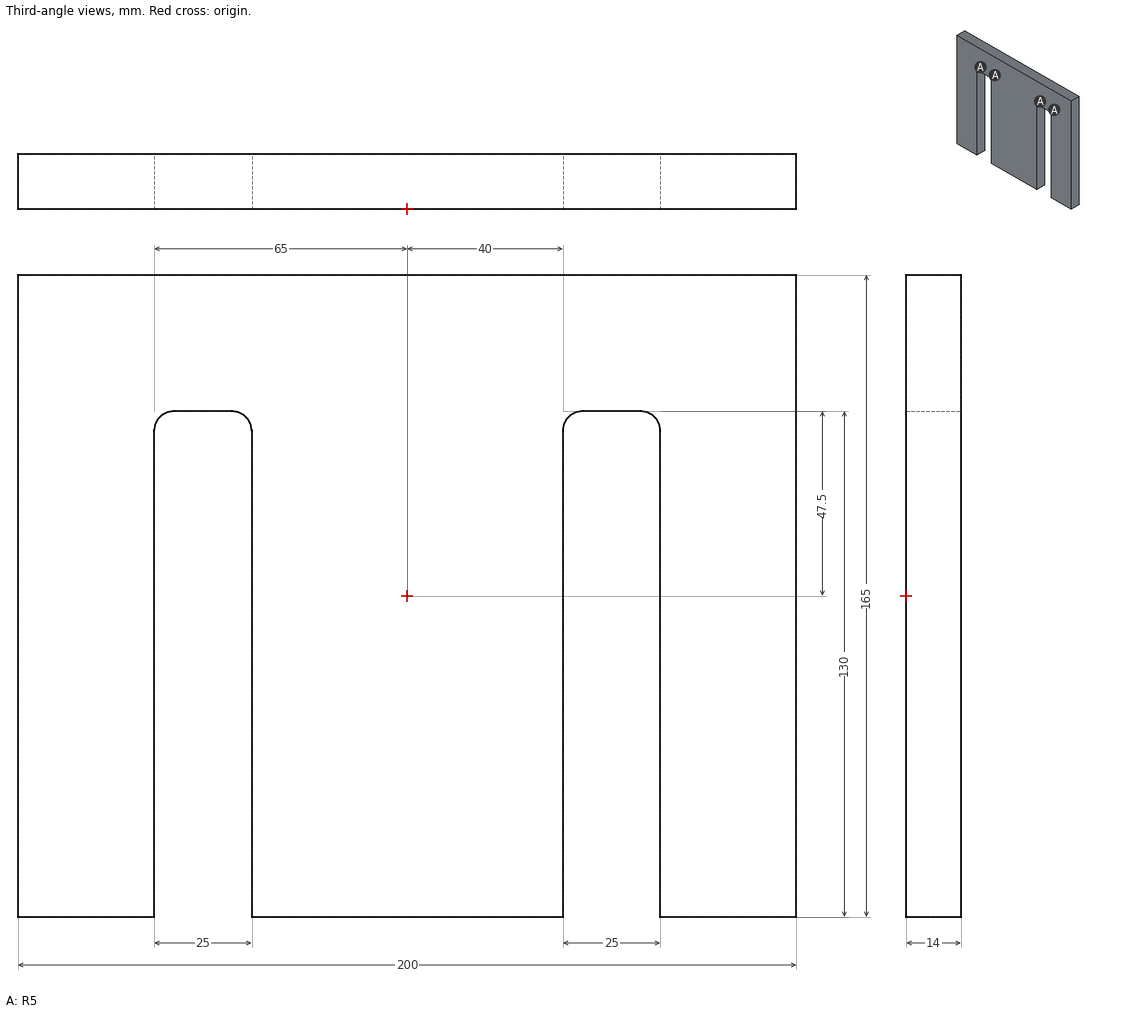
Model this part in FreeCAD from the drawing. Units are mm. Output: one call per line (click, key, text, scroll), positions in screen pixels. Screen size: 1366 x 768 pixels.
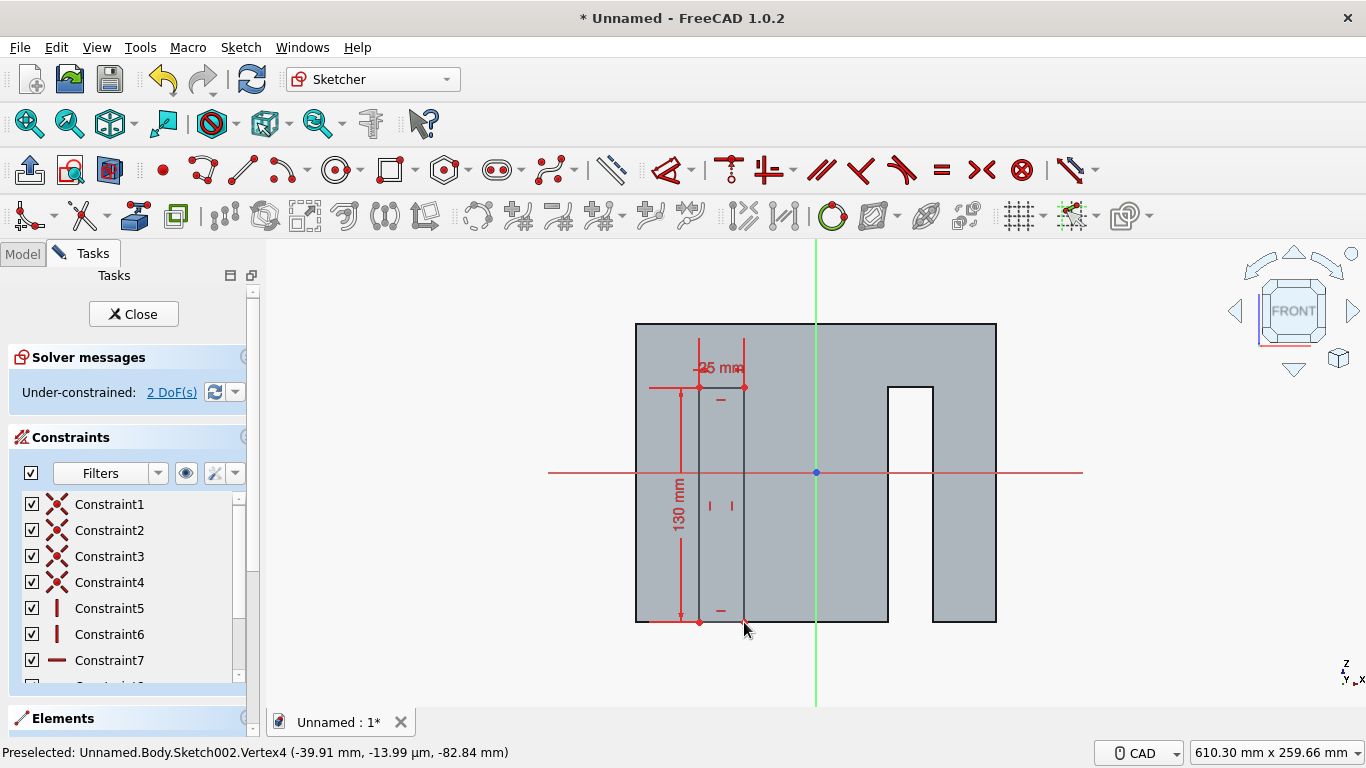
click(666, 170)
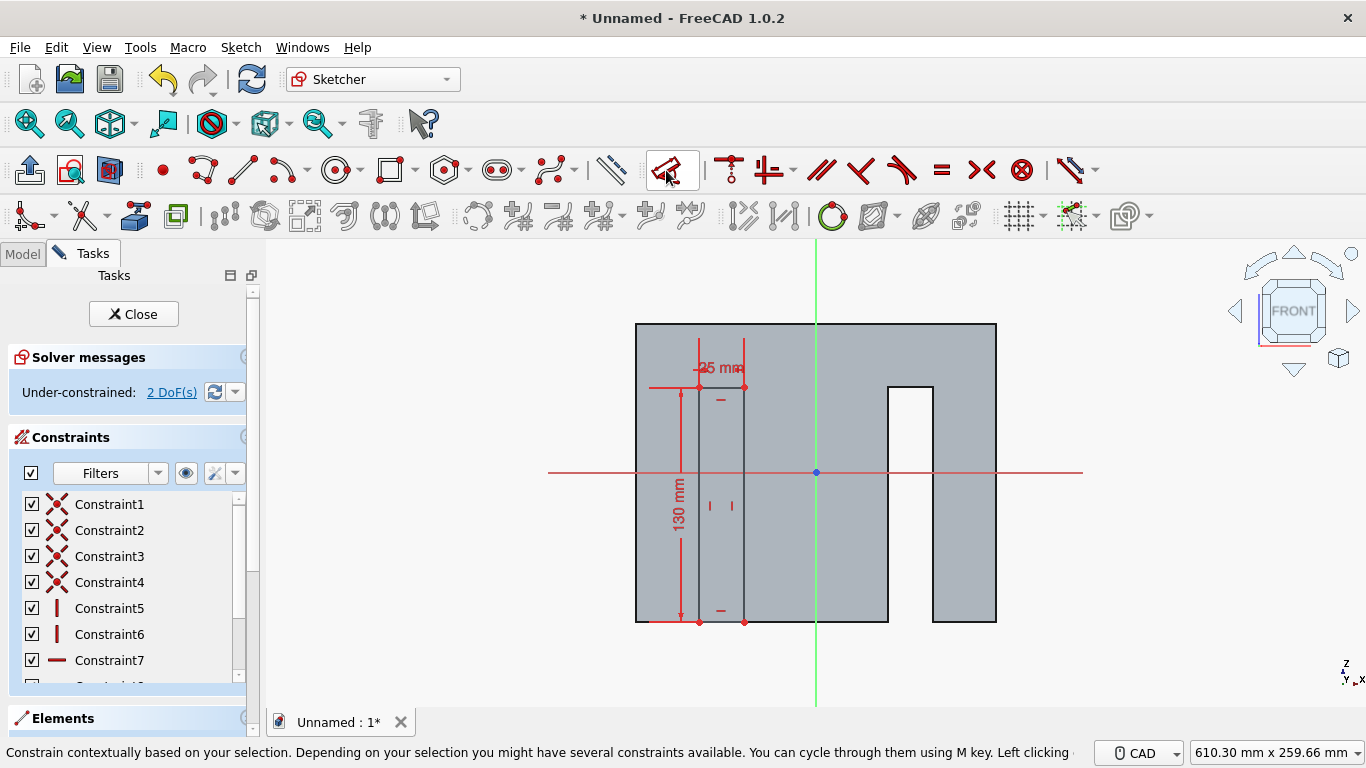
click(699, 388)
click(758, 354)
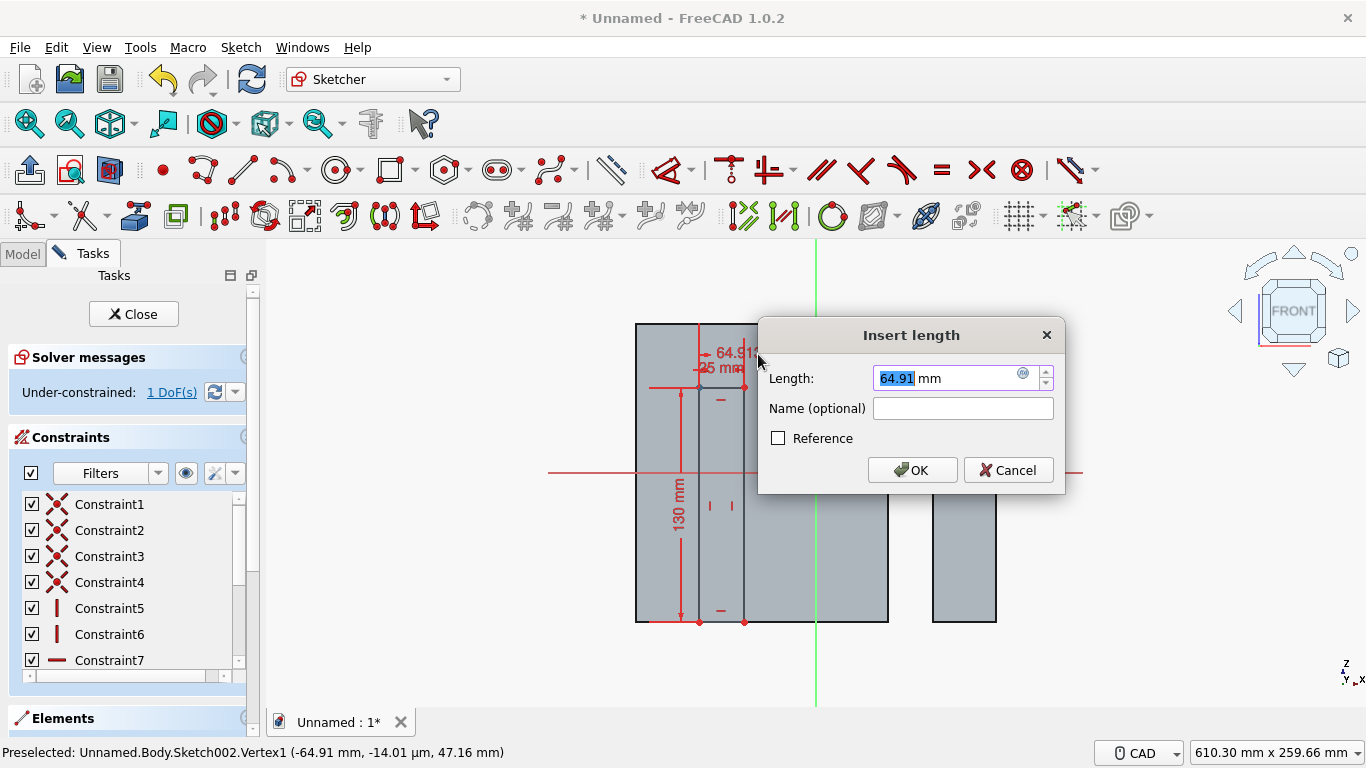
text(65)
key(Return)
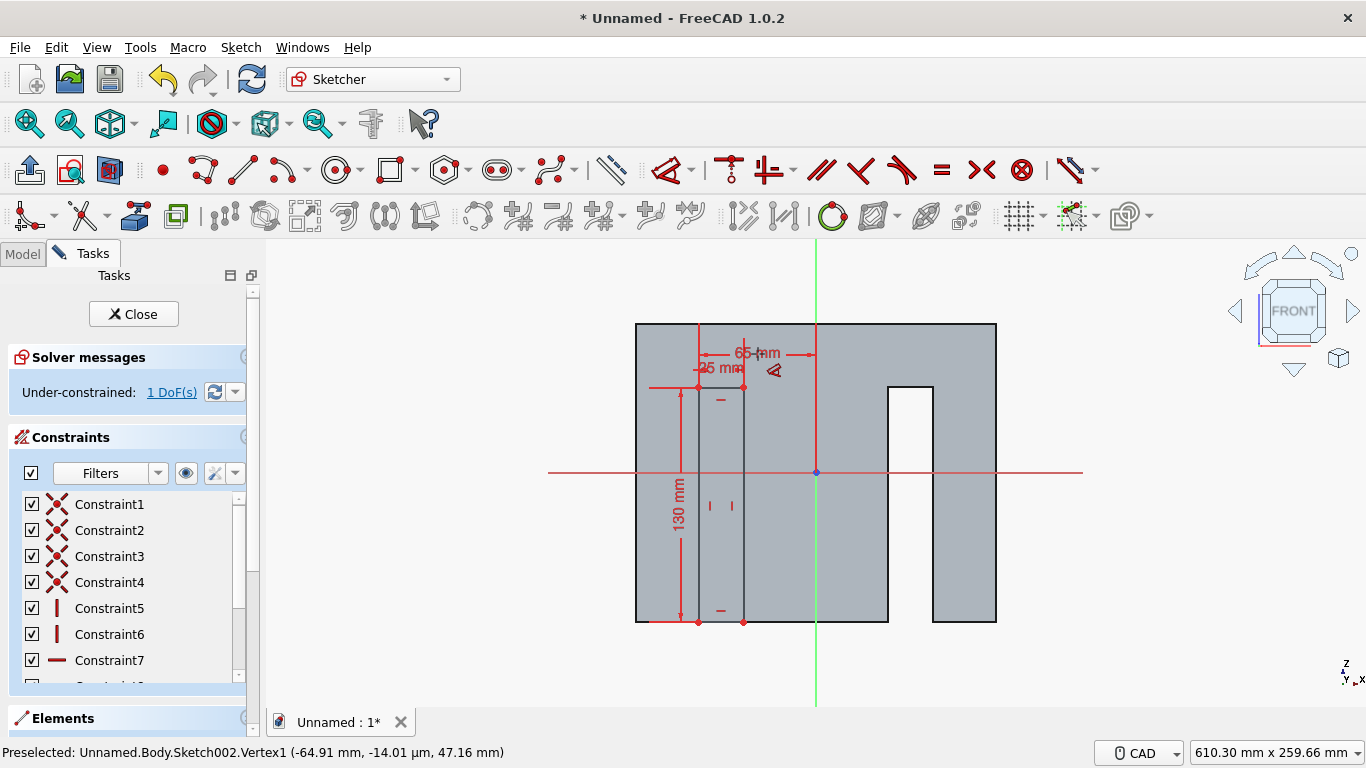
click(699, 388)
click(850, 430)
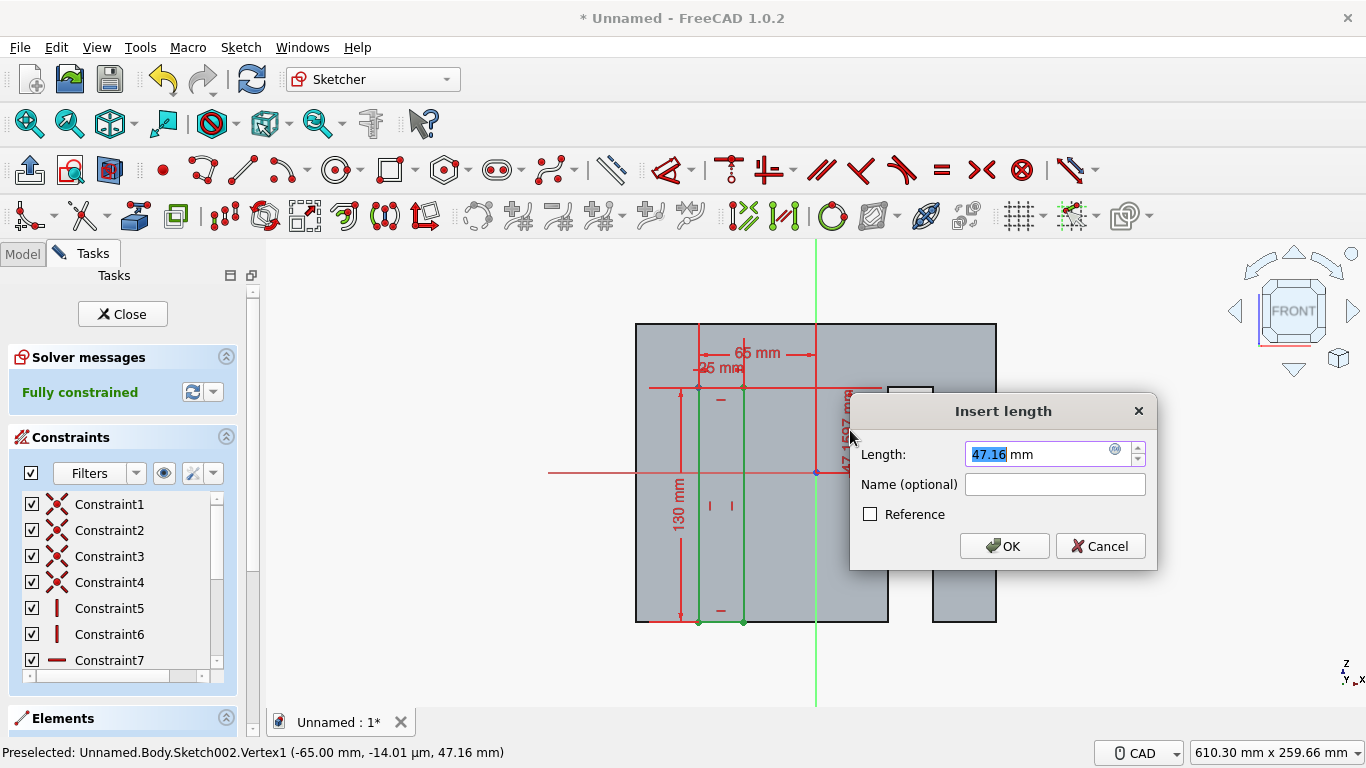
text(47.5)
key(Return)
key(Escape)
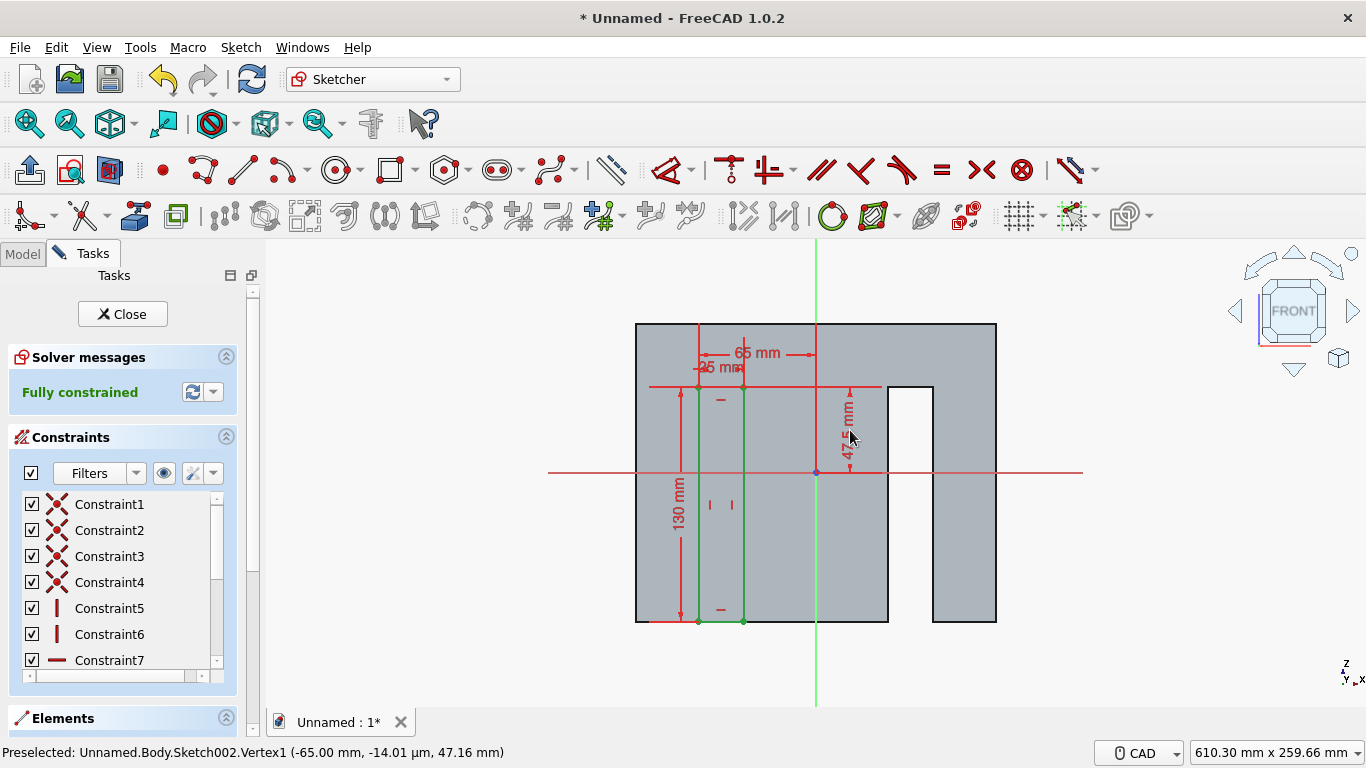
click(123, 314)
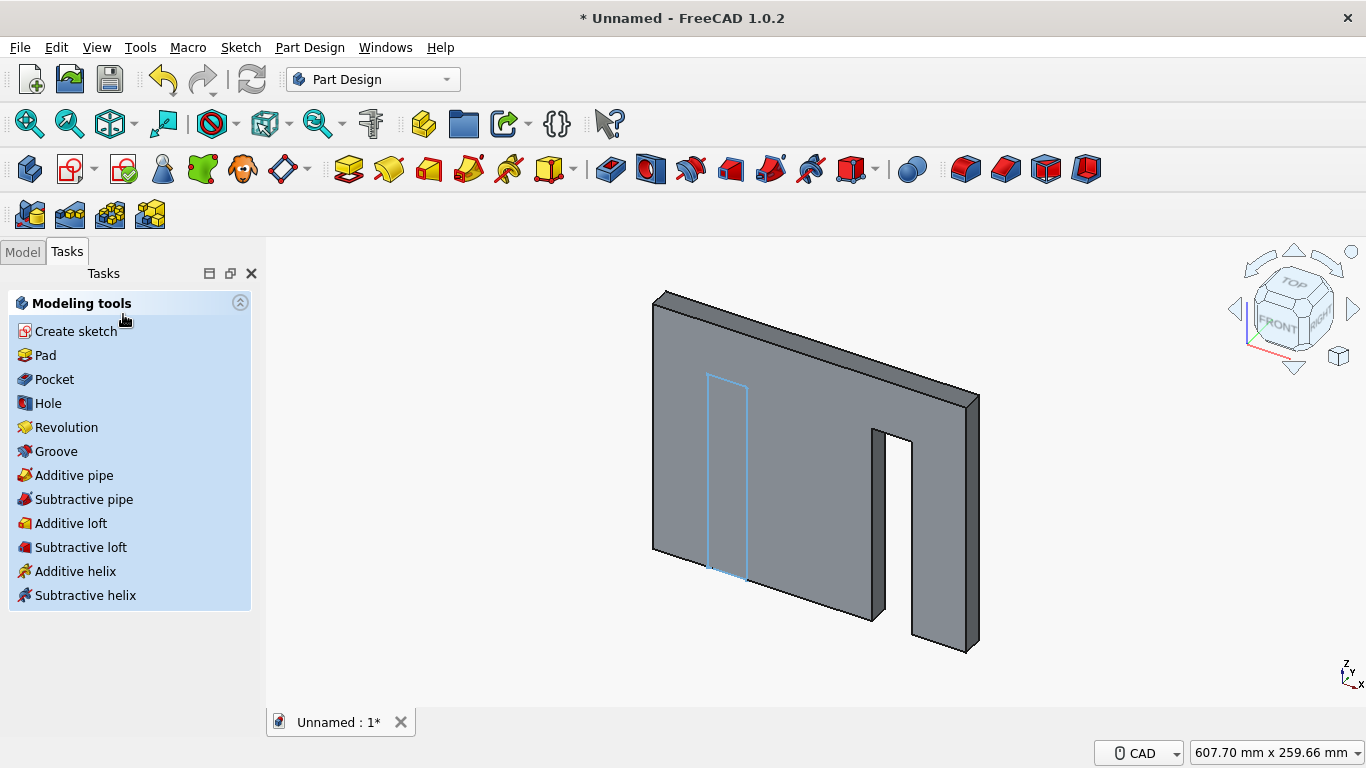
click(612, 170)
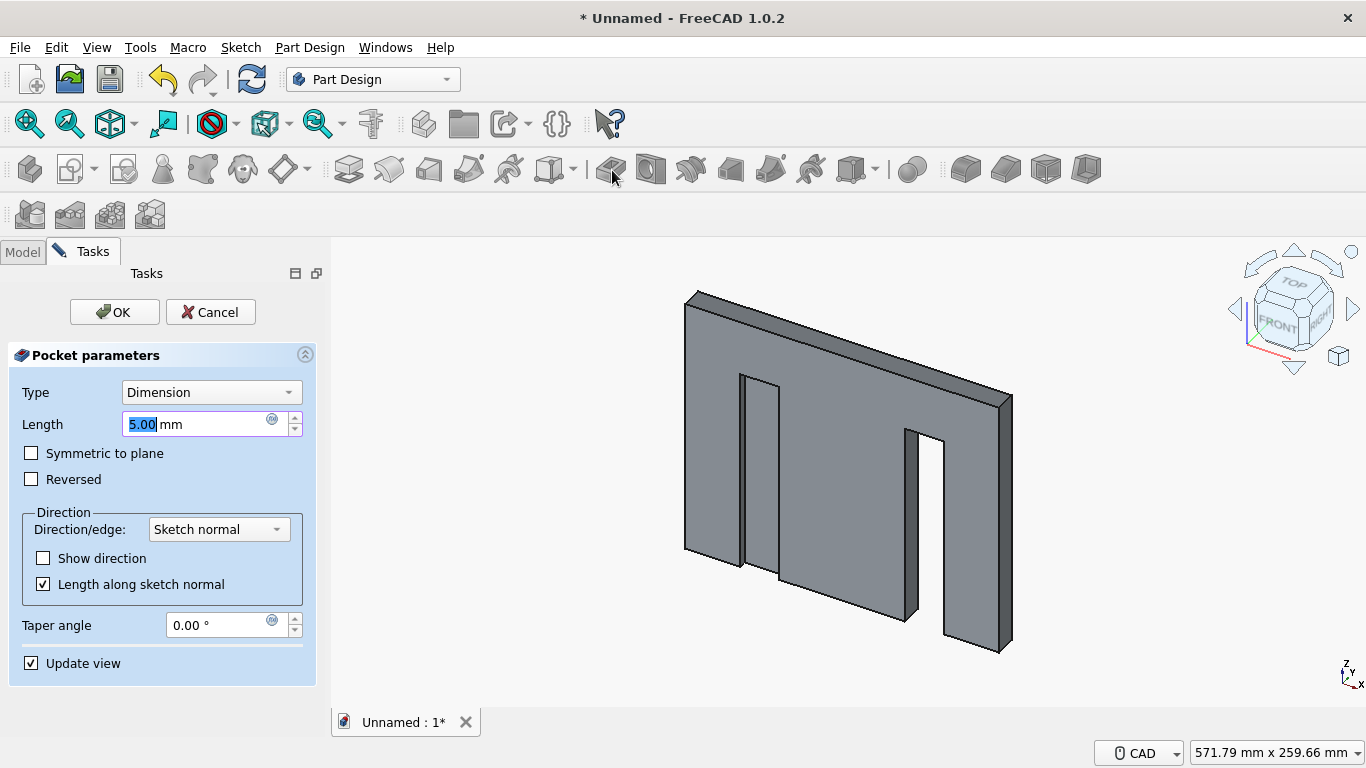
click(212, 392)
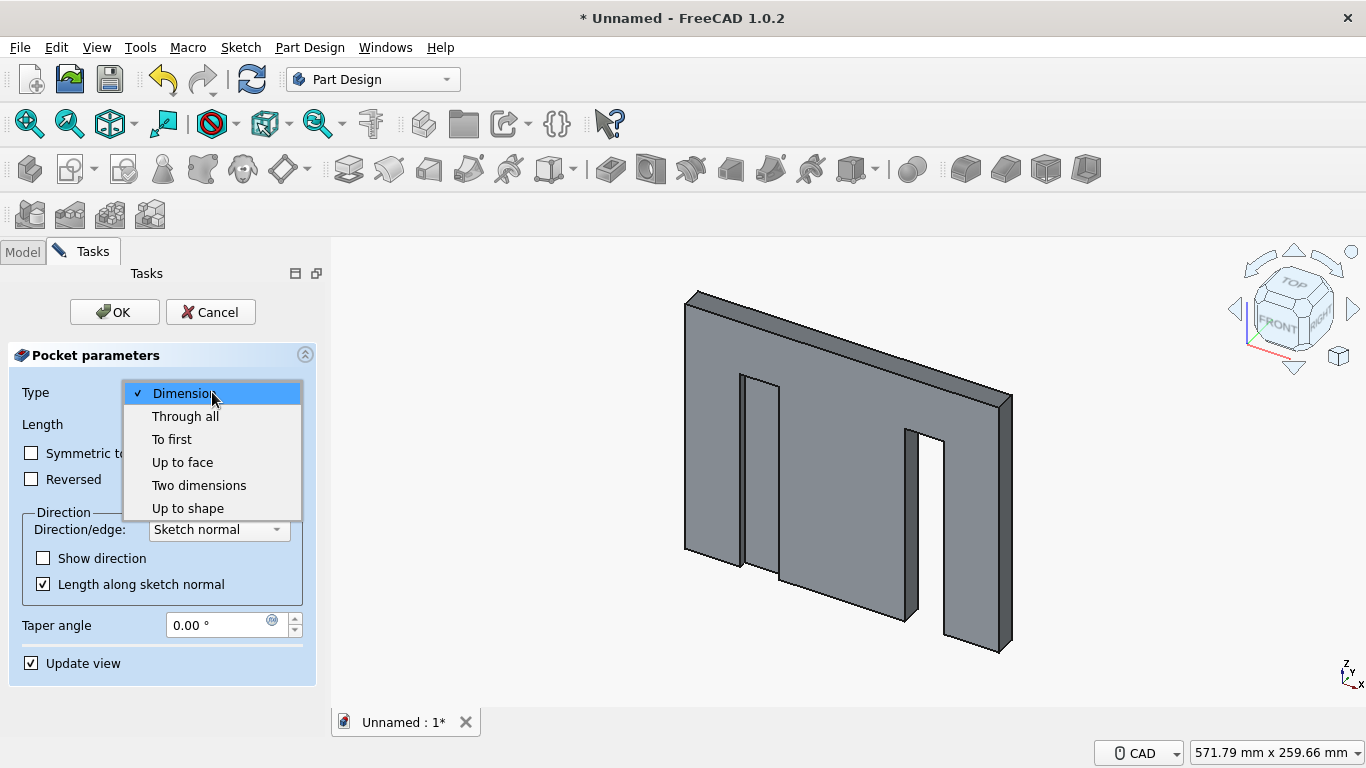
click(212, 440)